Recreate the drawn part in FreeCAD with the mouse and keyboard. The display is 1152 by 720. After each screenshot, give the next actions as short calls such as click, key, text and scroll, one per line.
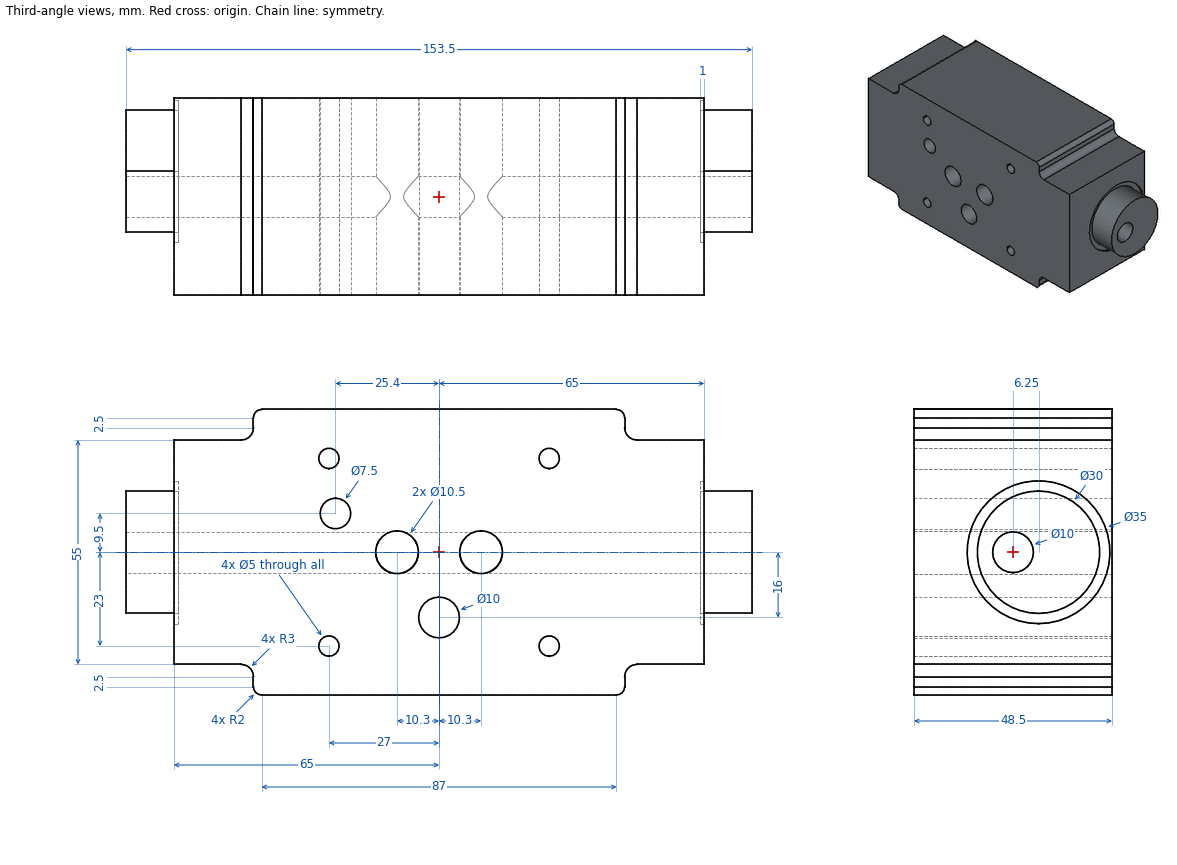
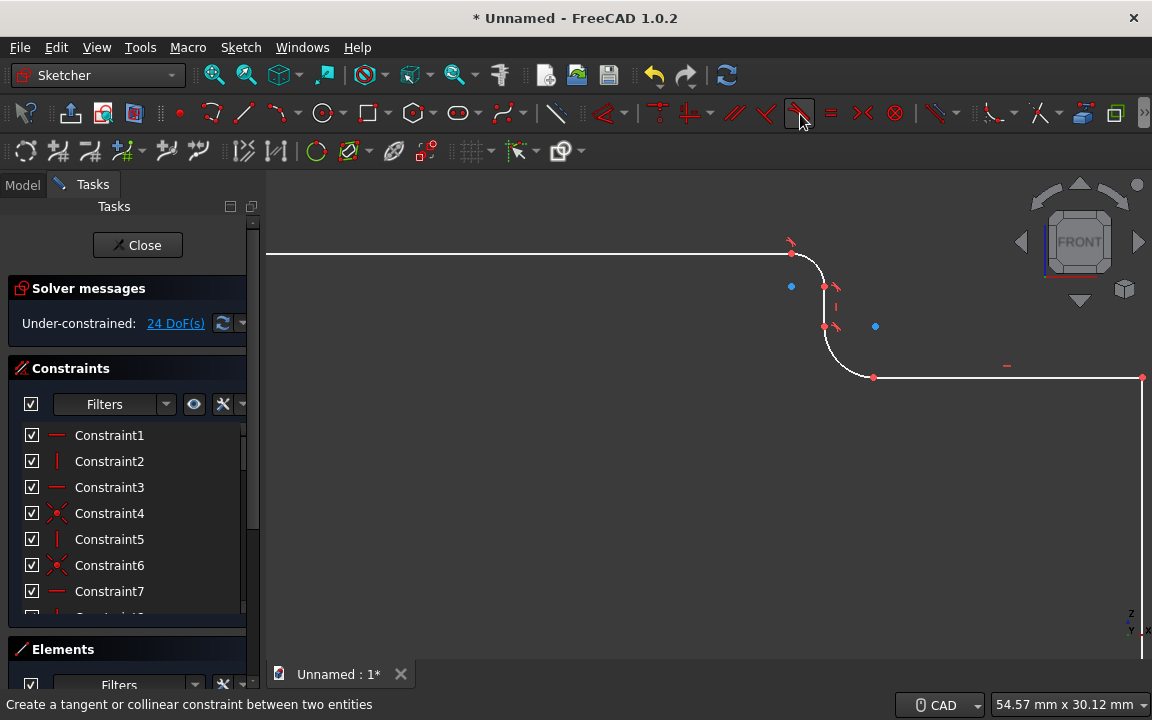
scroll(822, 282, down, 7)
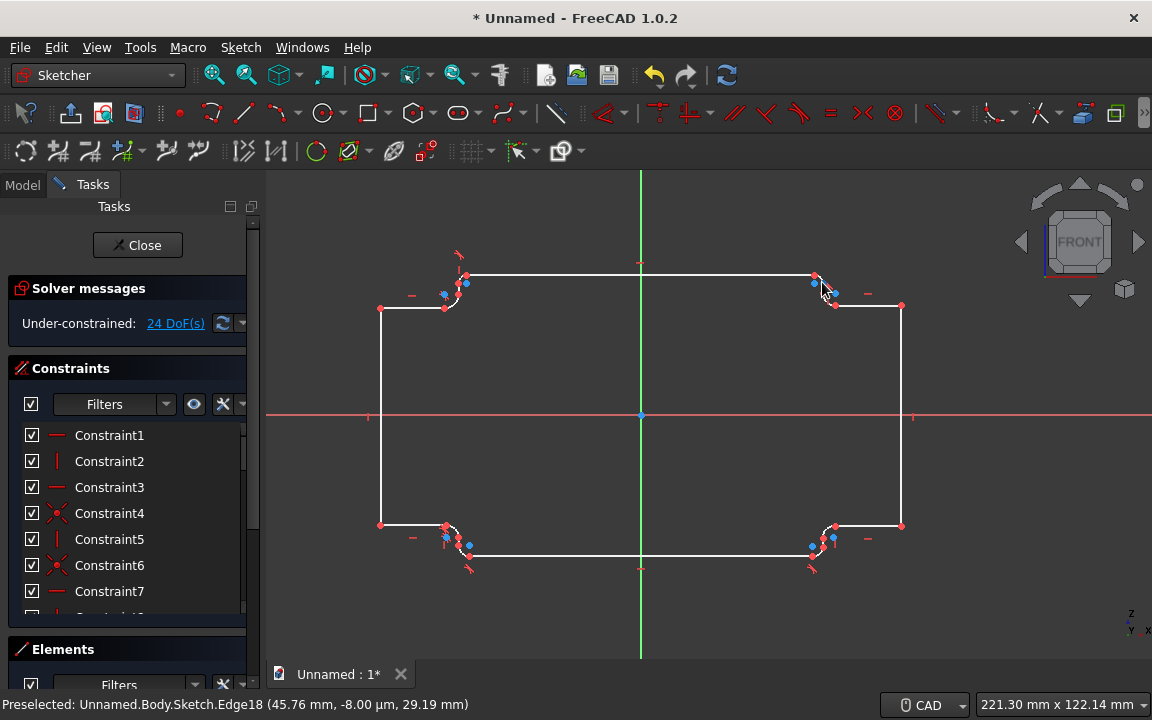
click(855, 306)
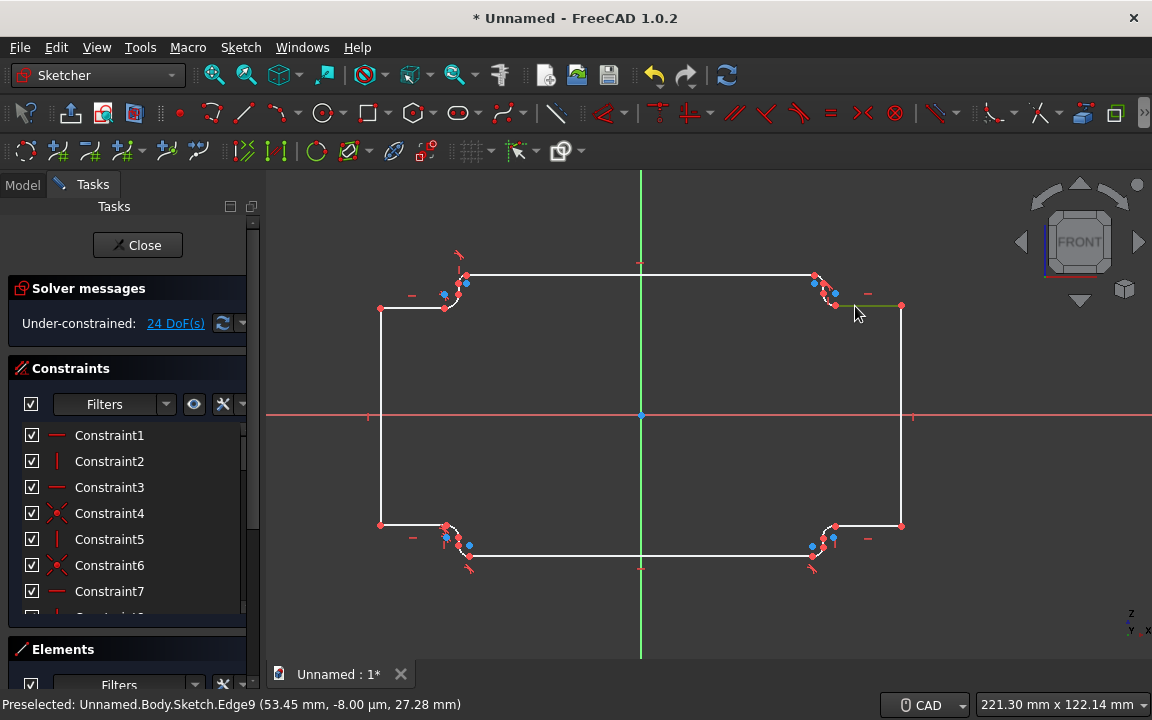
scroll(827, 302, up, 2)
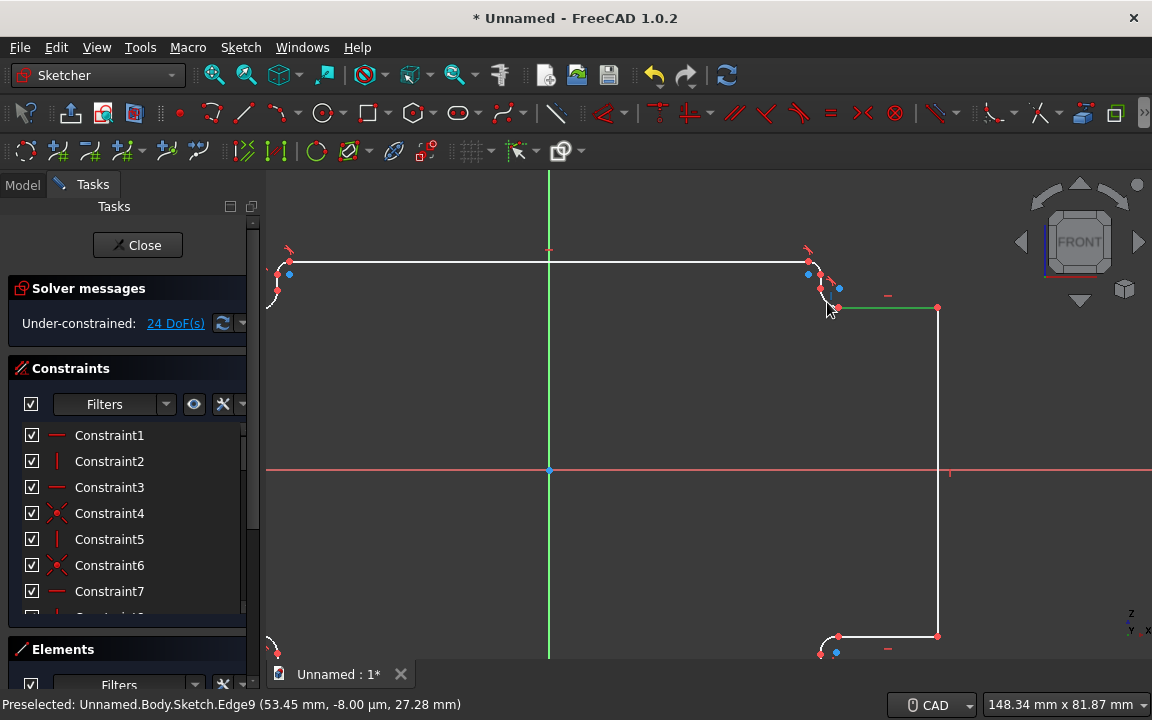
click(826, 302)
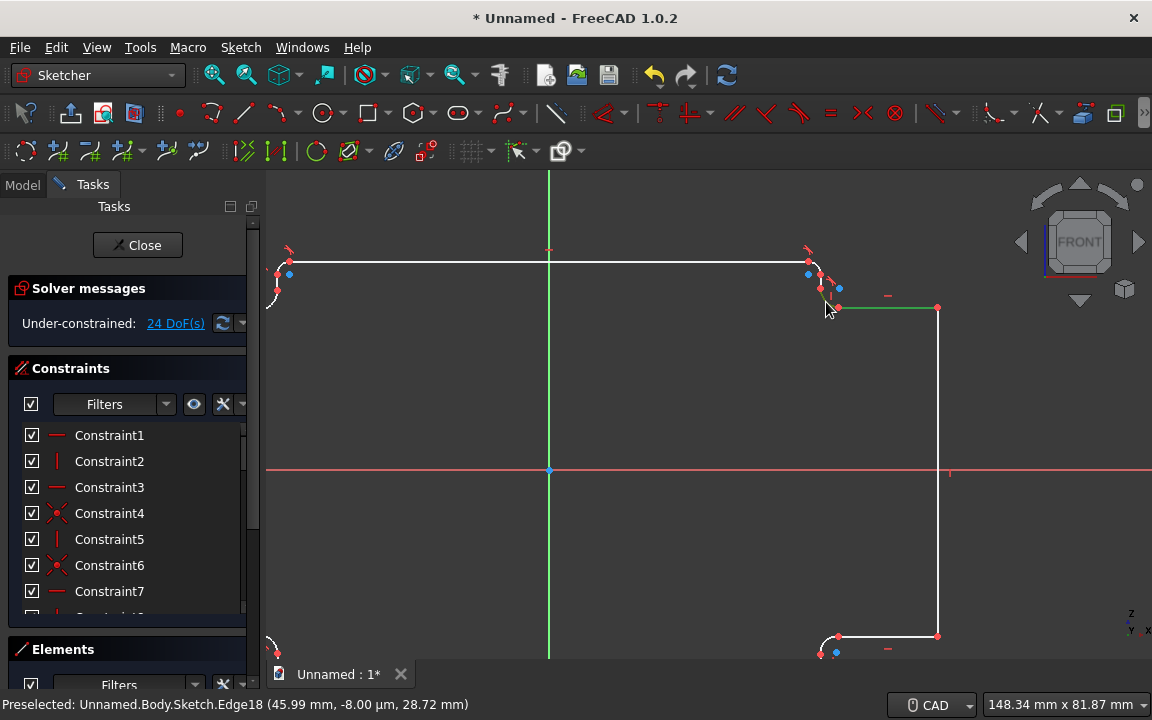
click(800, 114)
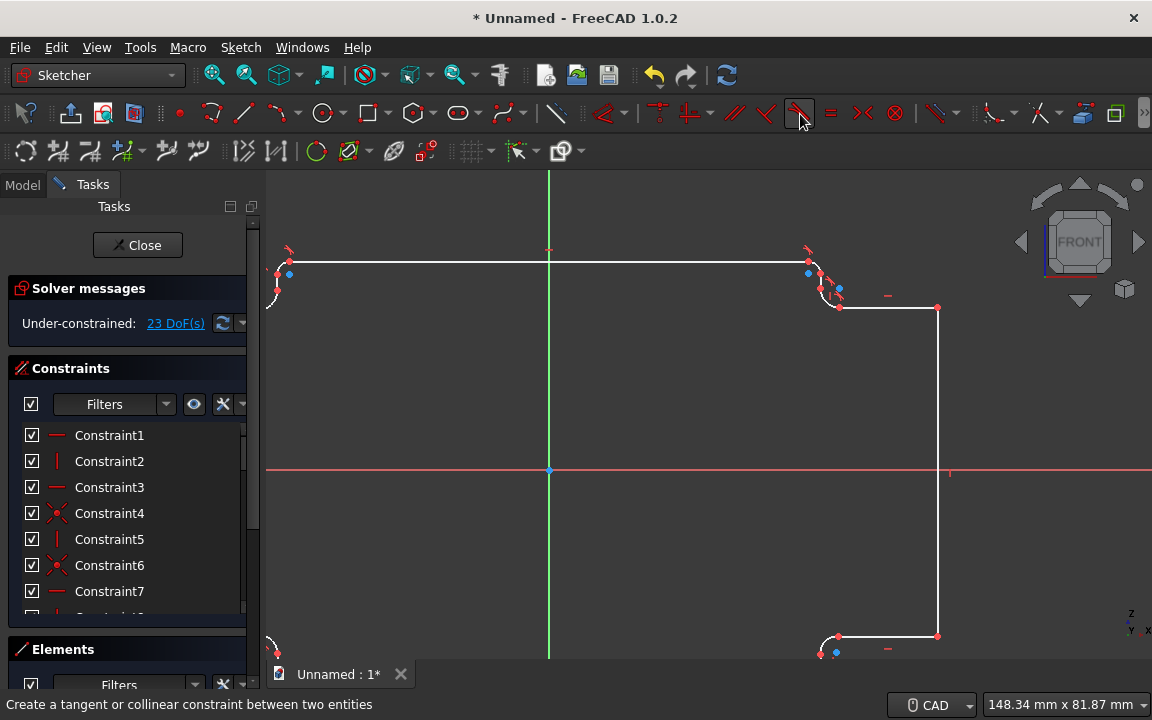
scroll(826, 301, down, 2)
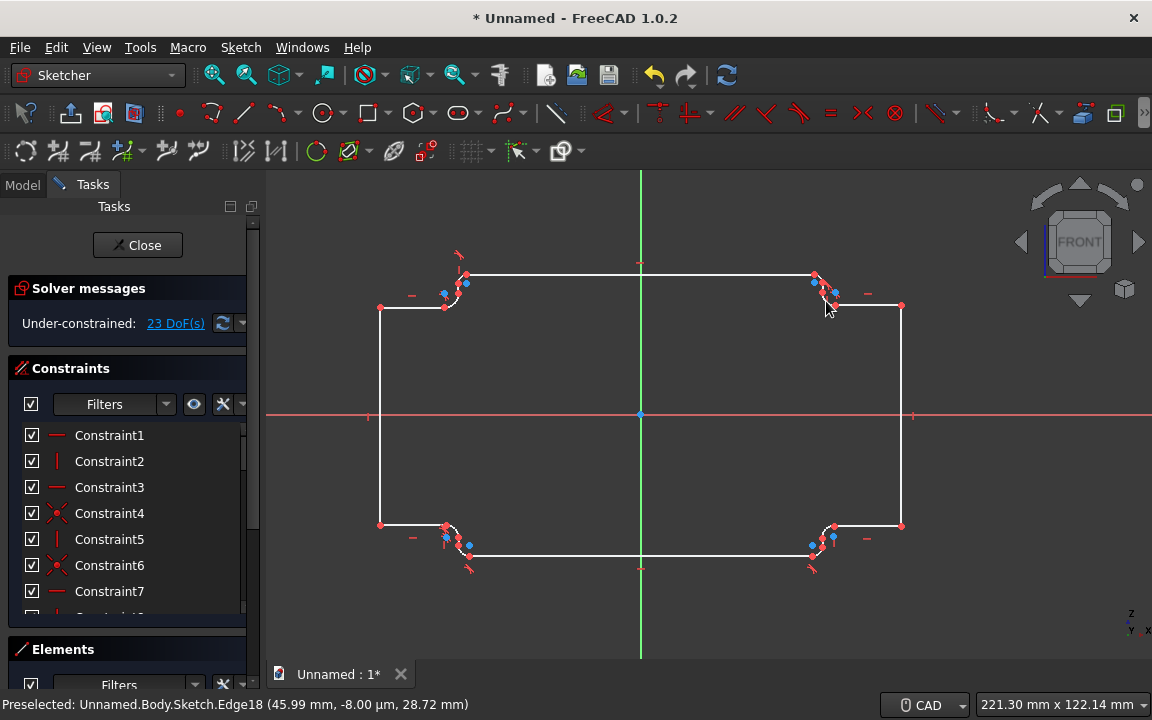
click(881, 526)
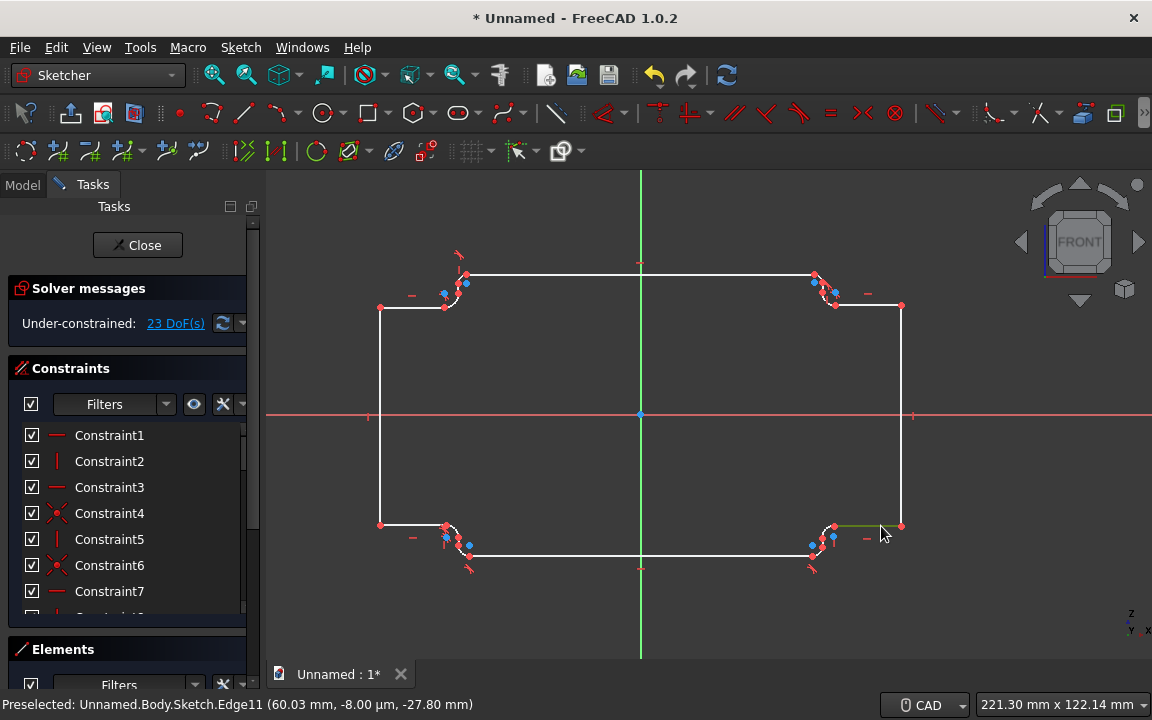
scroll(826, 529, up, 2)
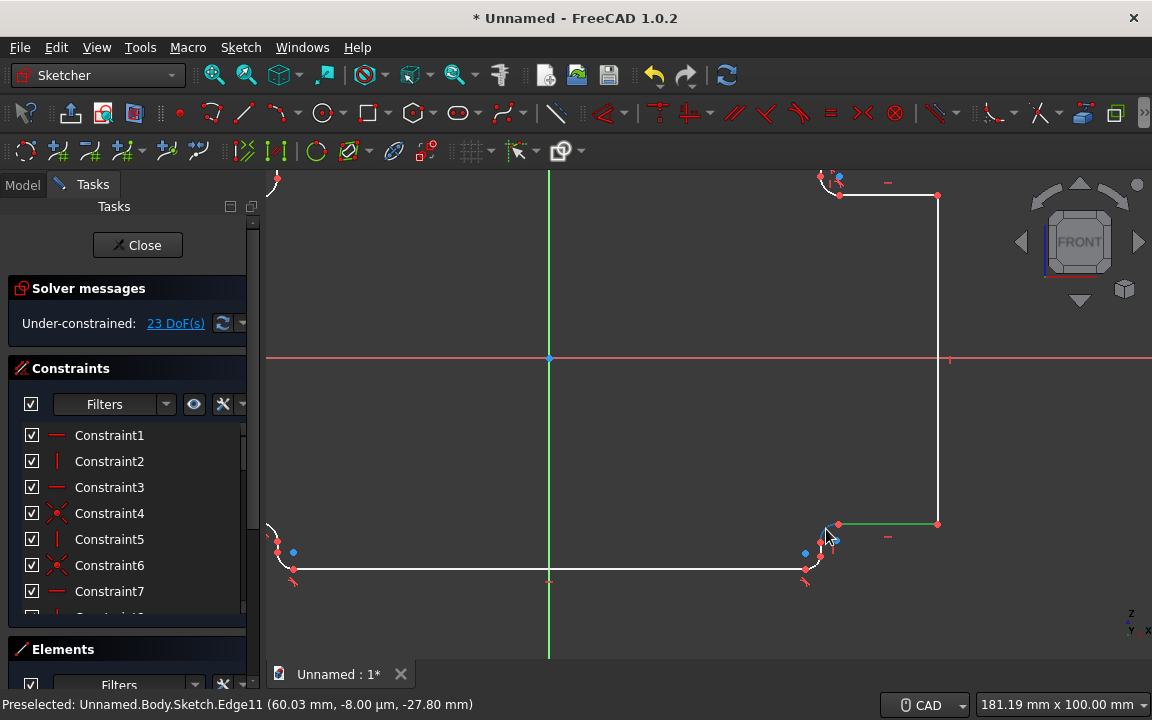
click(825, 529)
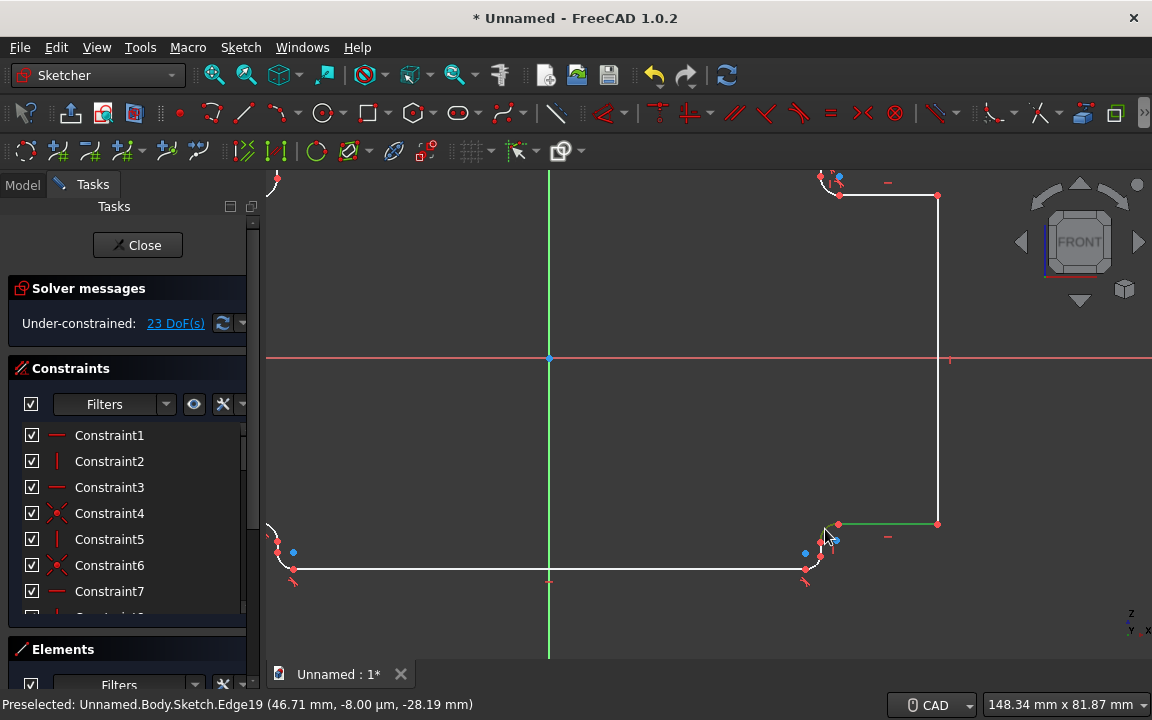
click(800, 114)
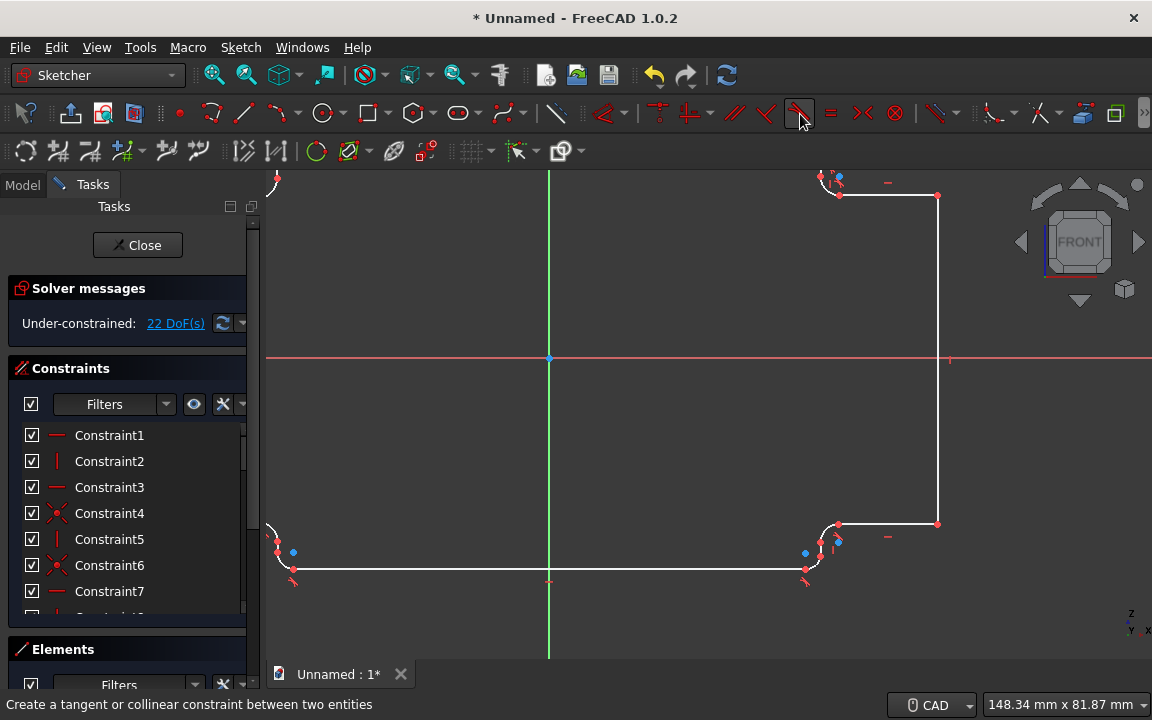
scroll(821, 549, up, 4)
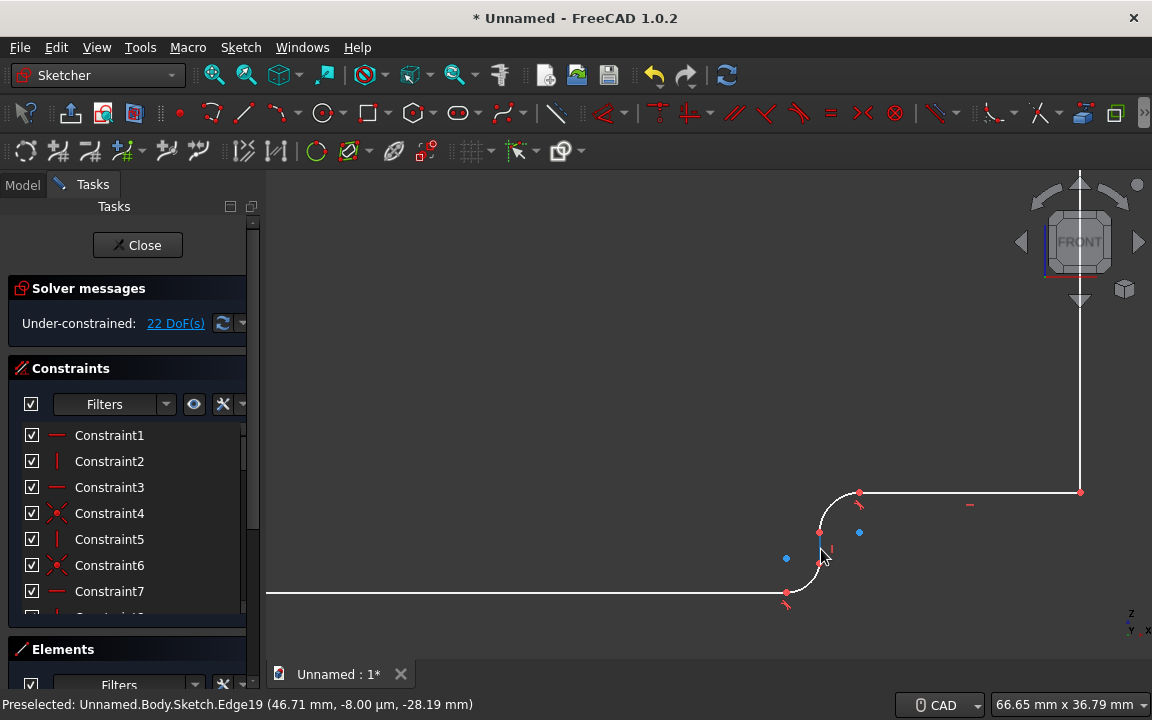
click(820, 548)